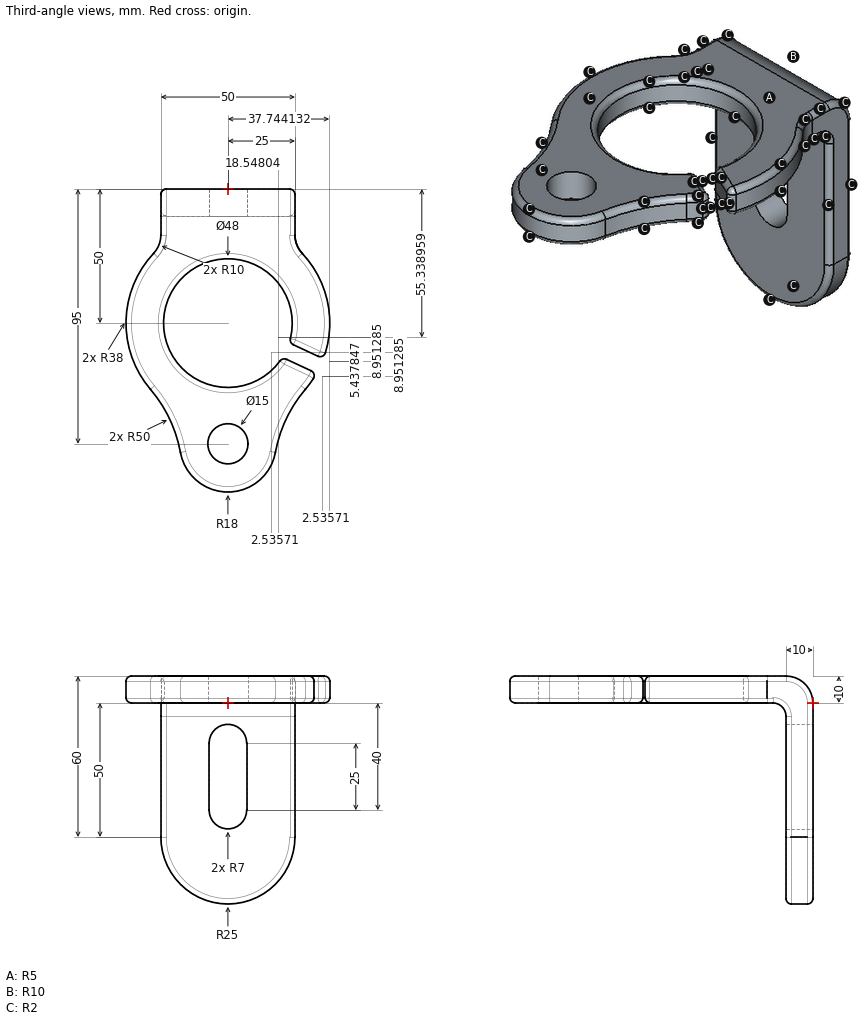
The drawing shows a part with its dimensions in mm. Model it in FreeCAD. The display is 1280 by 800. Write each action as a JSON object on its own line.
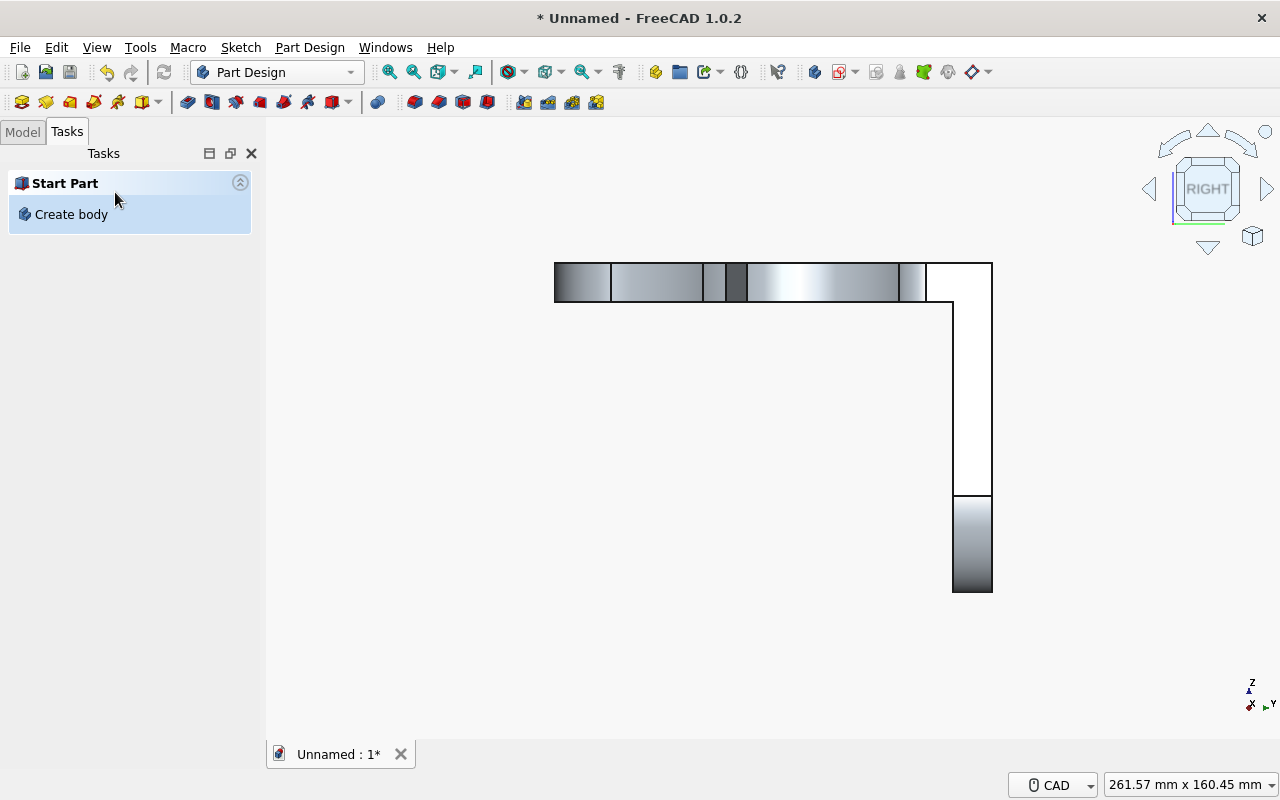
{"action": "key", "text": "5"}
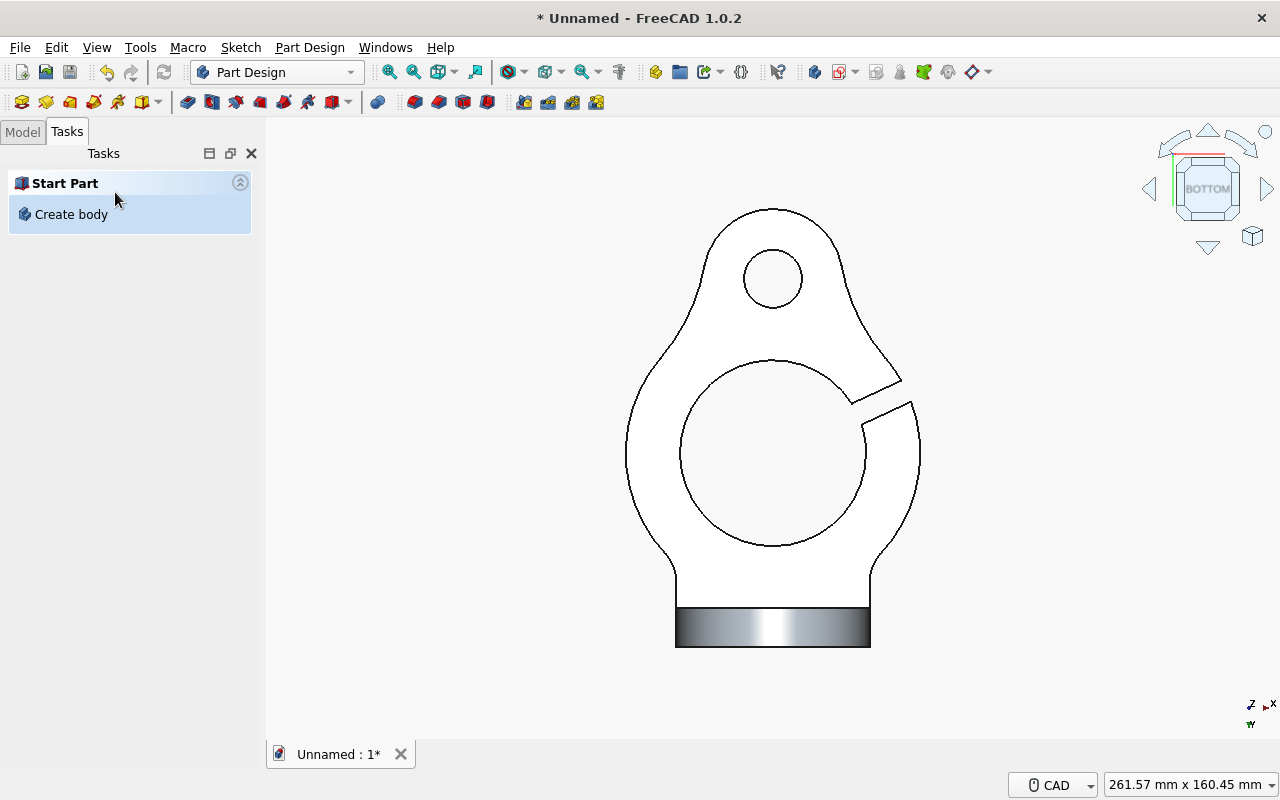
{"action": "key", "text": "4"}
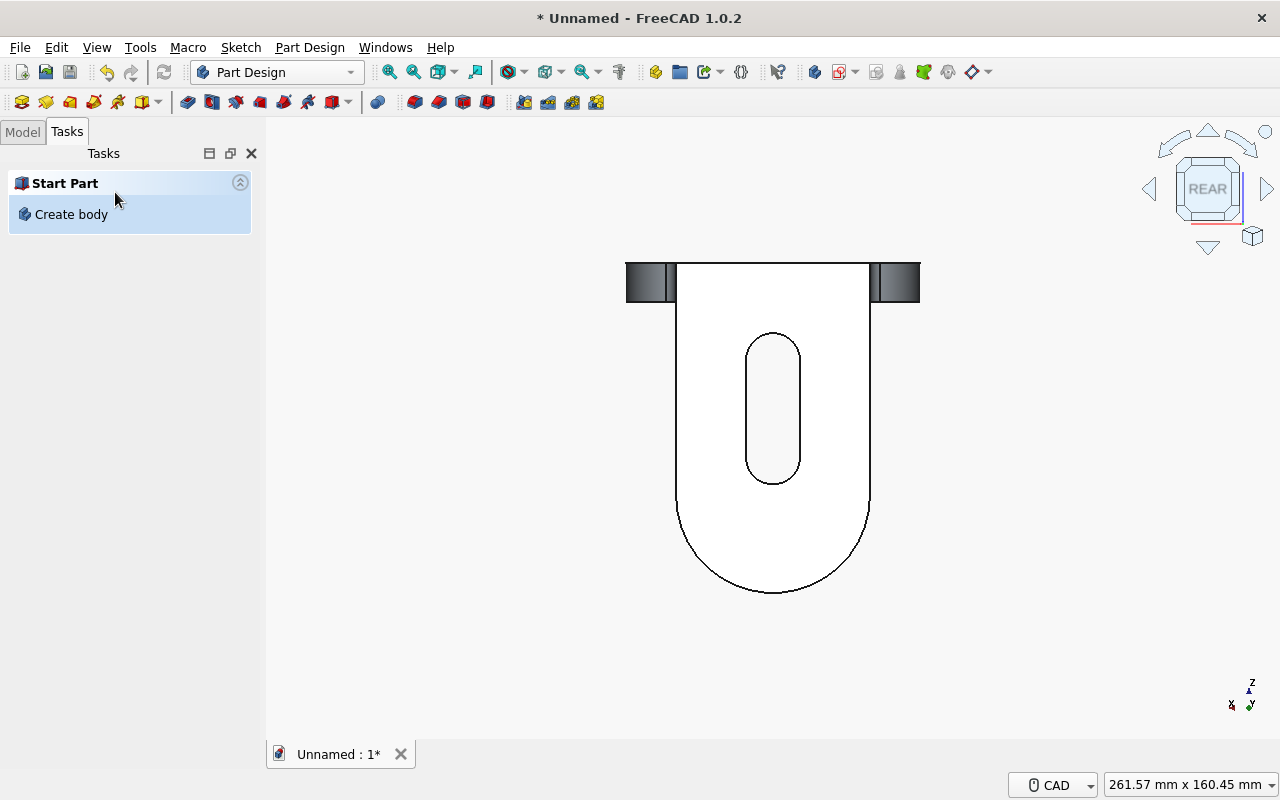
{"action": "key", "text": "6"}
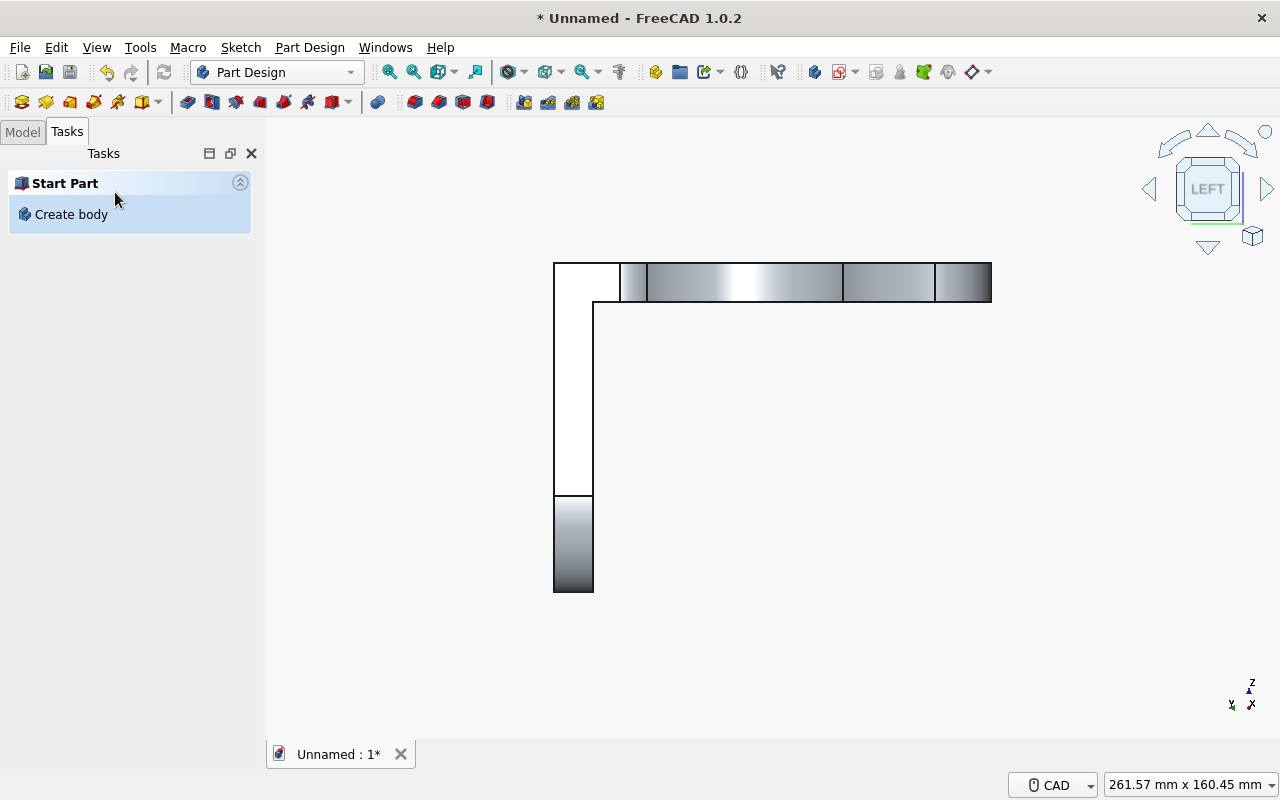
{"action": "key", "text": "v 3"}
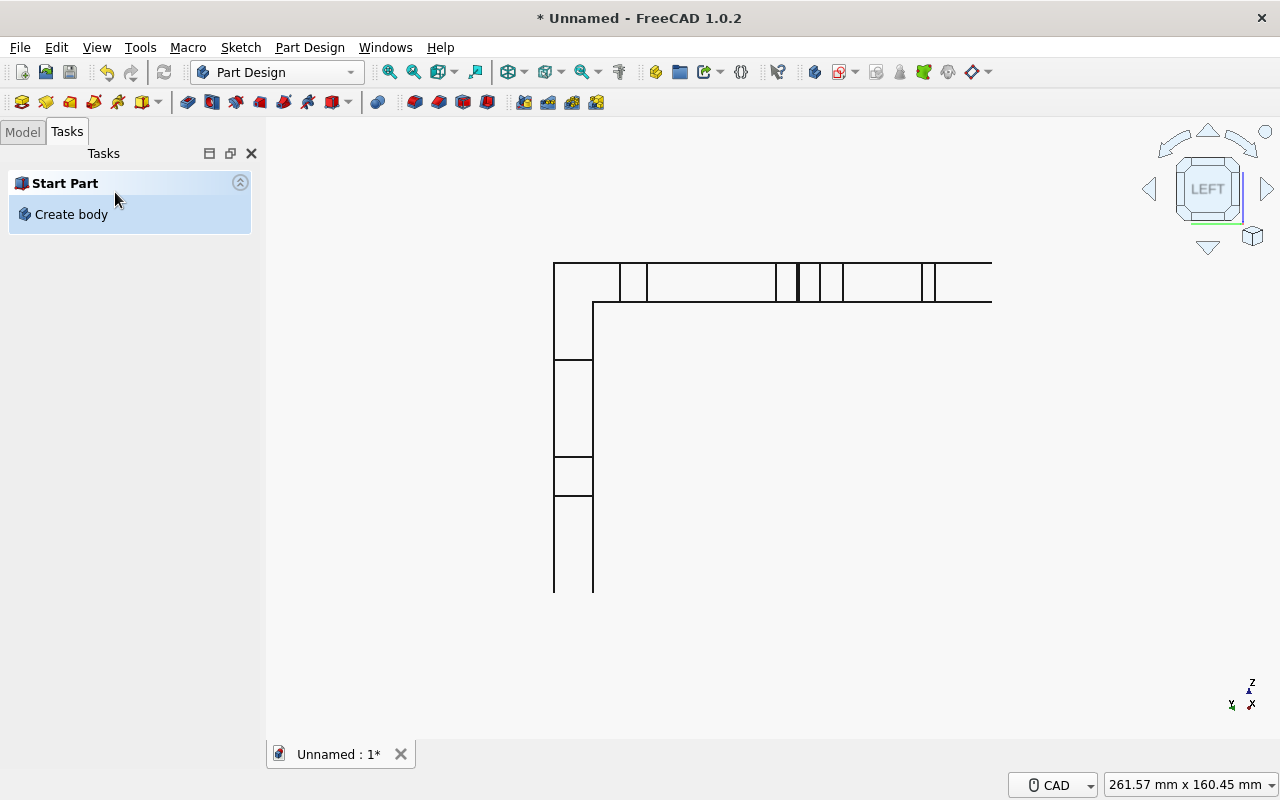
{"action": "key", "text": "0"}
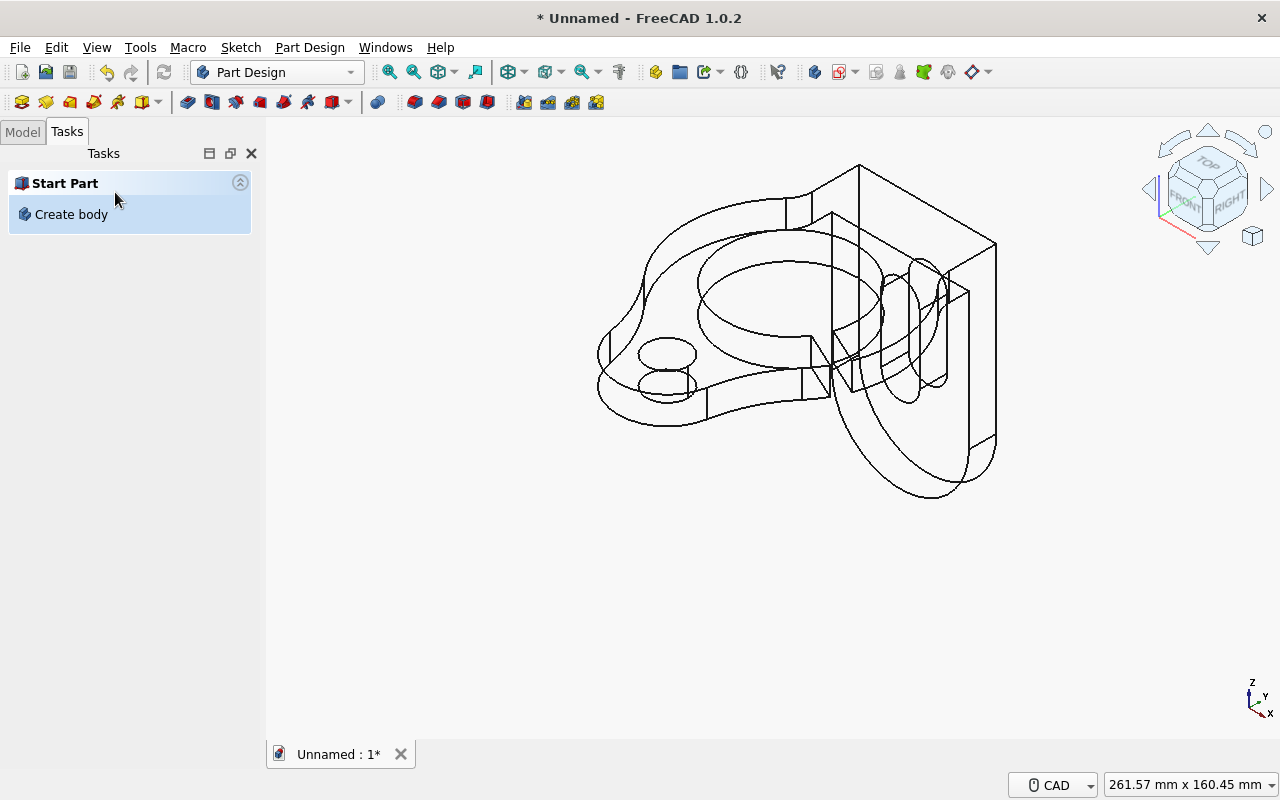
{"action": "left_click", "coordinate": [900, 251]}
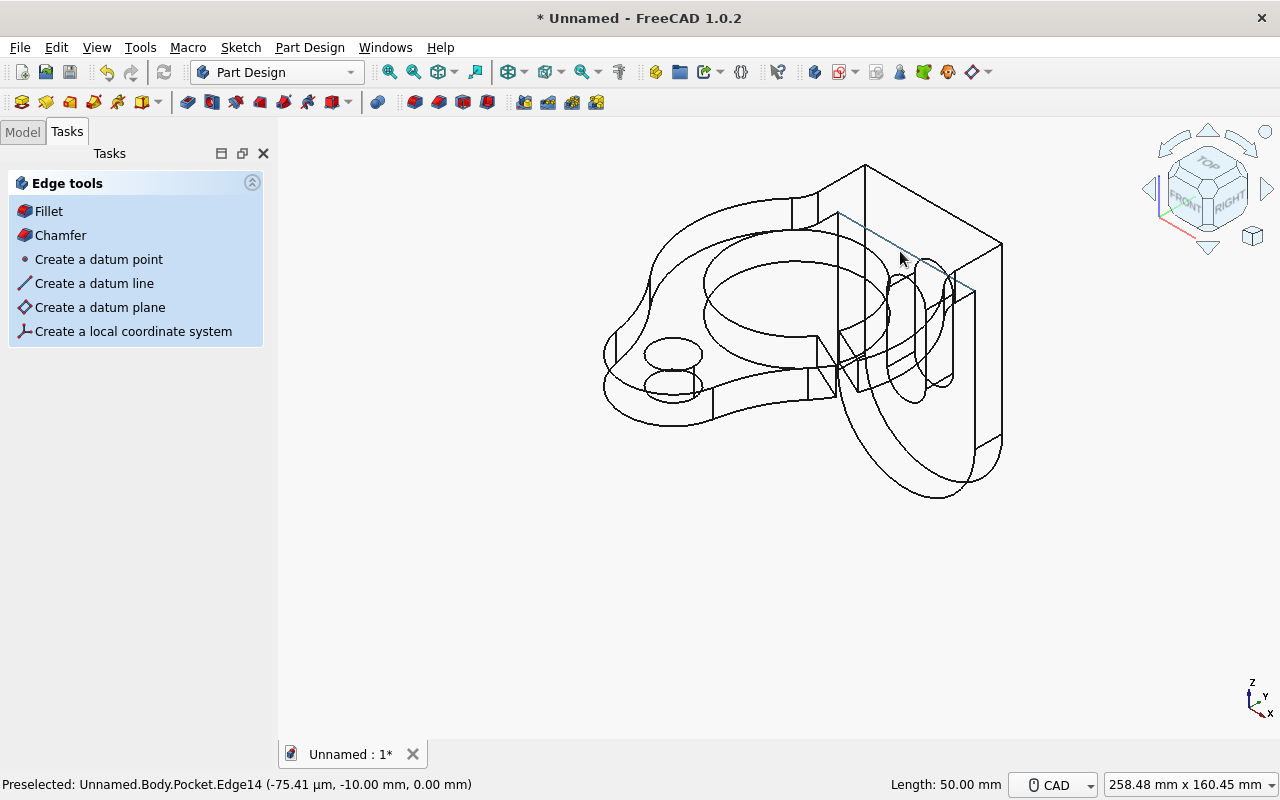
{"action": "key", "text": "v 1"}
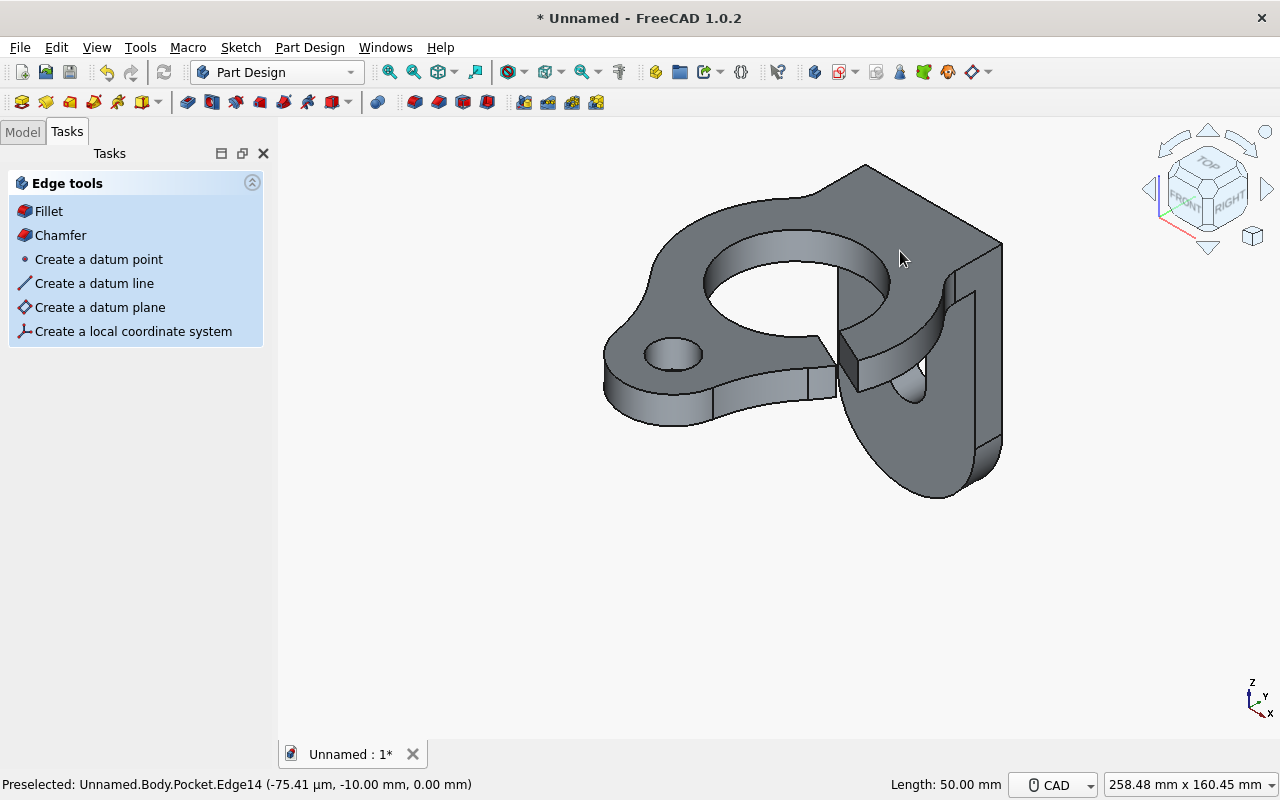
{"action": "left_click", "coordinate": [416, 102]}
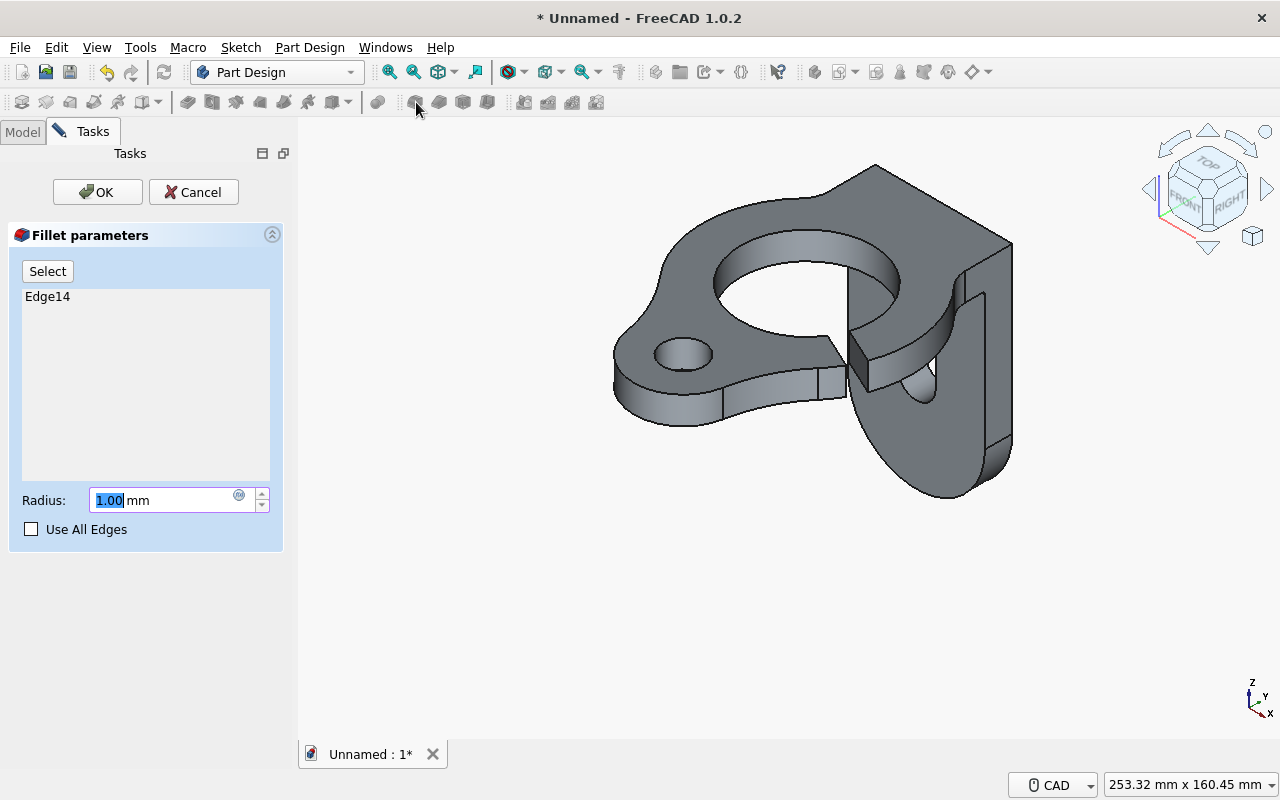
{"action": "type", "text": "5"}
{"action": "key", "text": "Tab"}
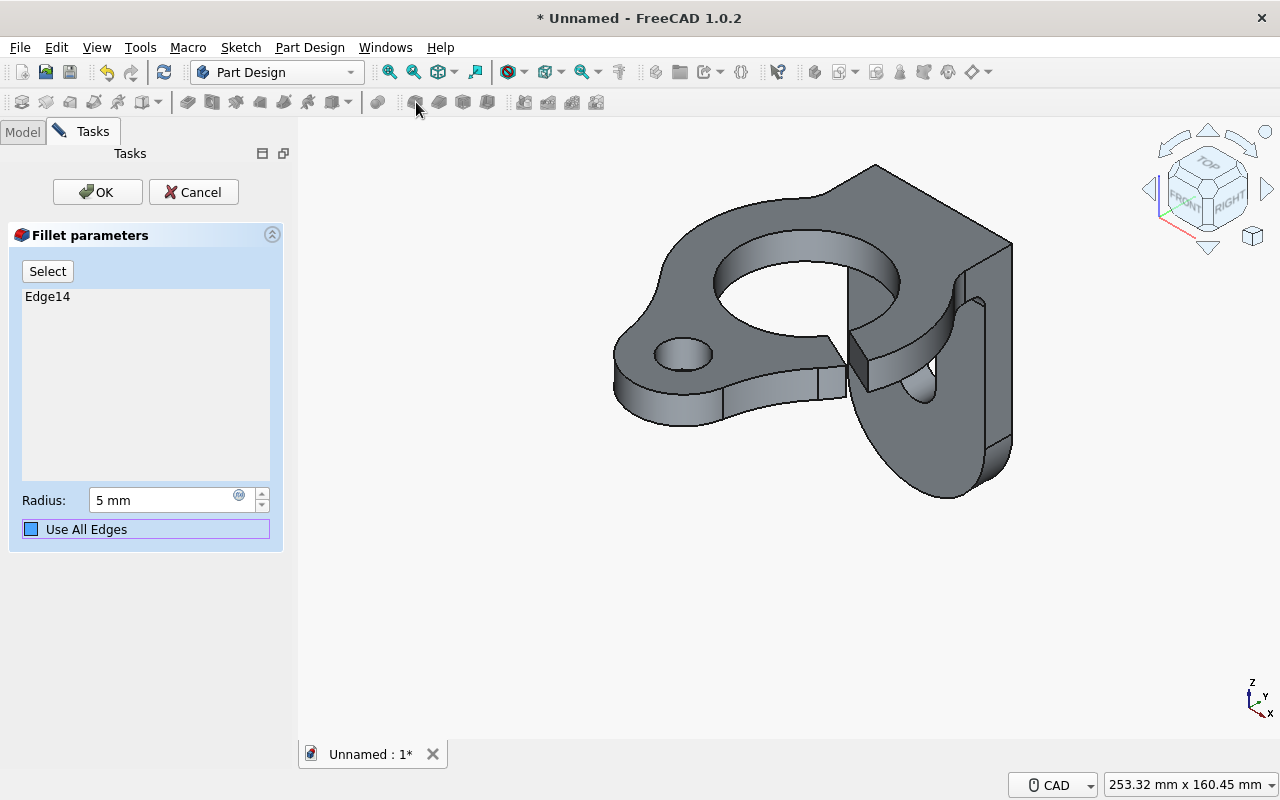
{"action": "left_click", "coordinate": [98, 192]}